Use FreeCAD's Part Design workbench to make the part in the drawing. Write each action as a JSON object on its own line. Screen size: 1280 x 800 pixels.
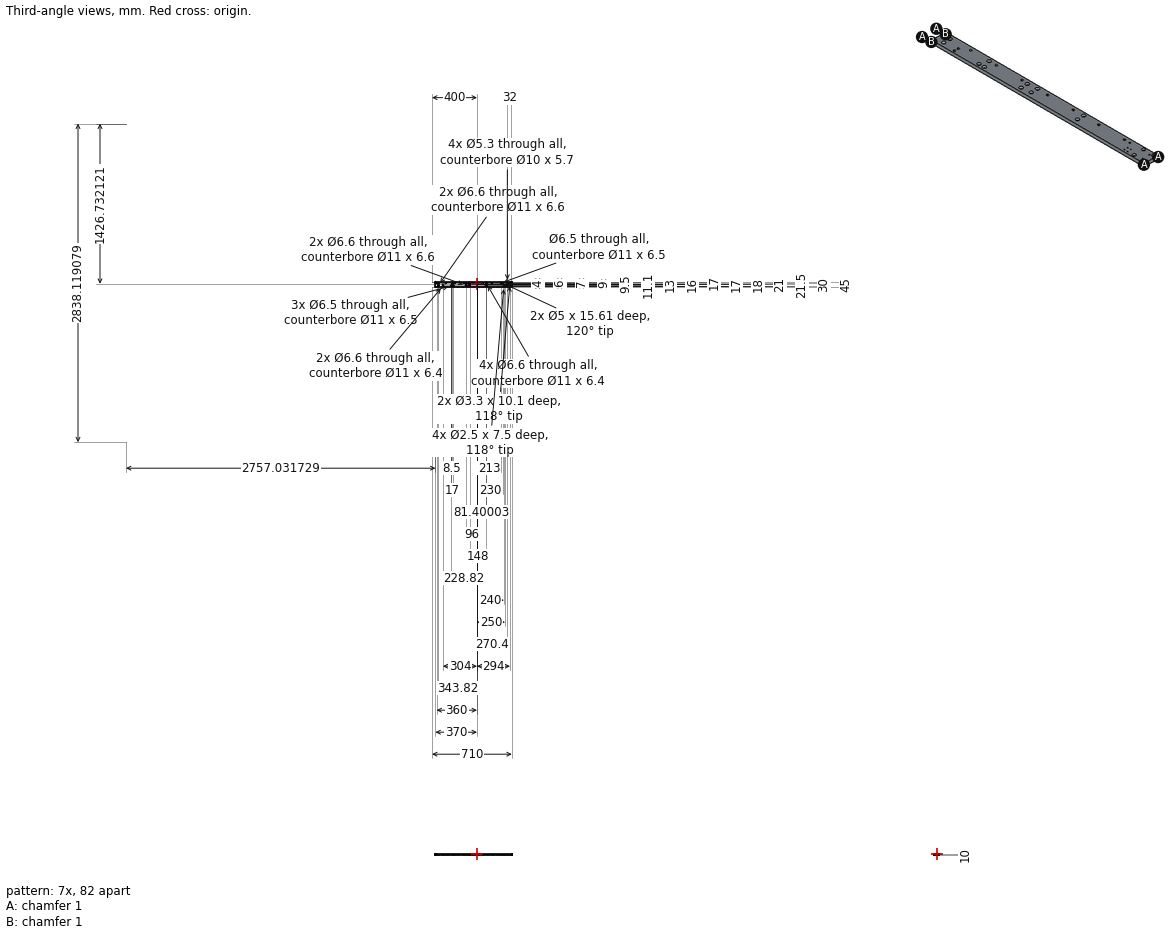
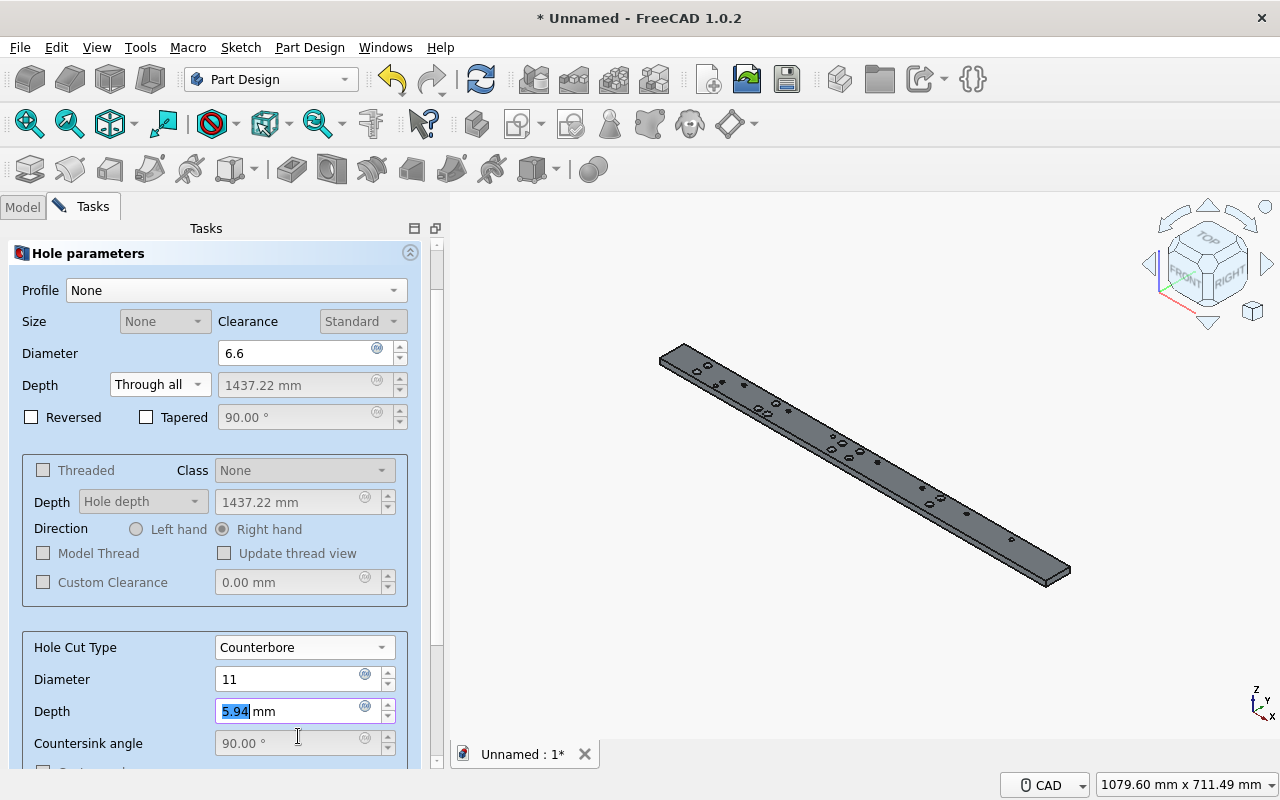
{"action": "type", "text": "6.4"}
{"action": "key", "text": "Tab"}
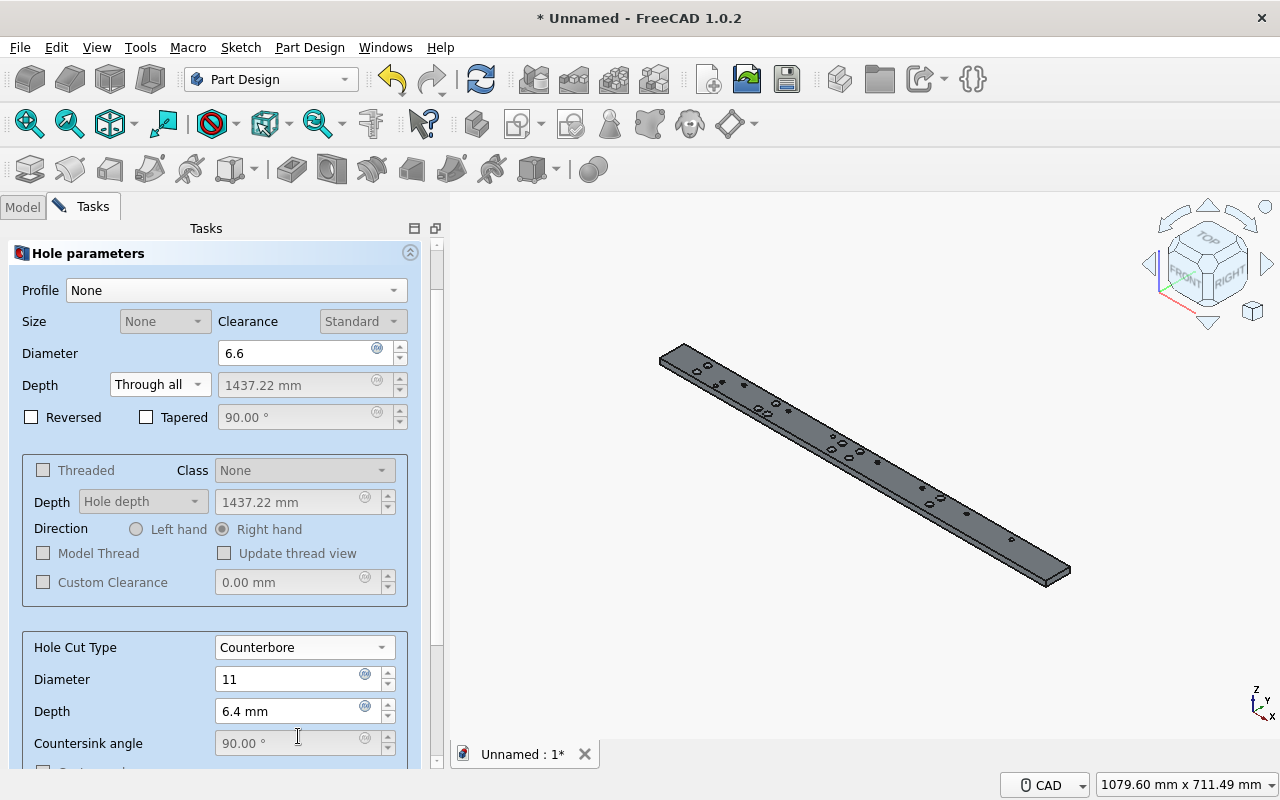
{"action": "scroll", "coordinate": [437, 503], "scroll_direction": "up", "scroll_amount": 2}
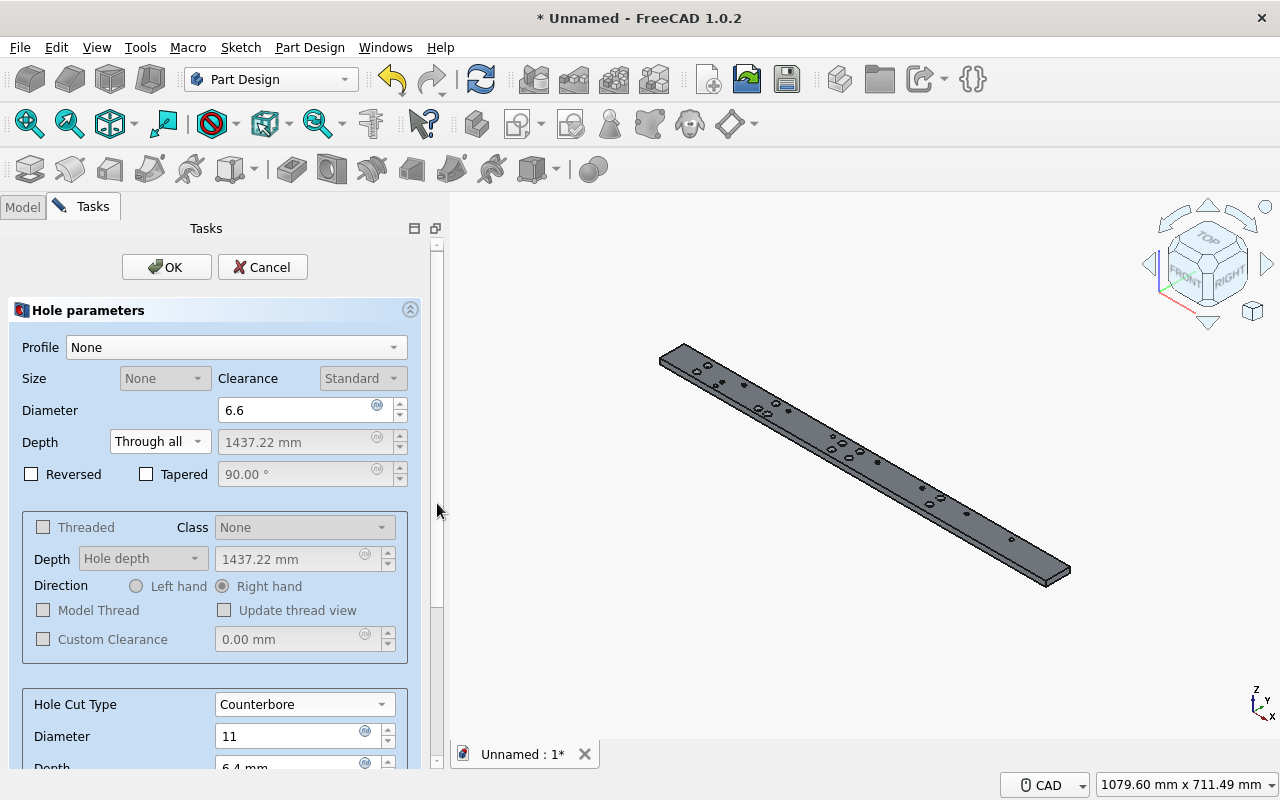
{"action": "left_click", "coordinate": [167, 267]}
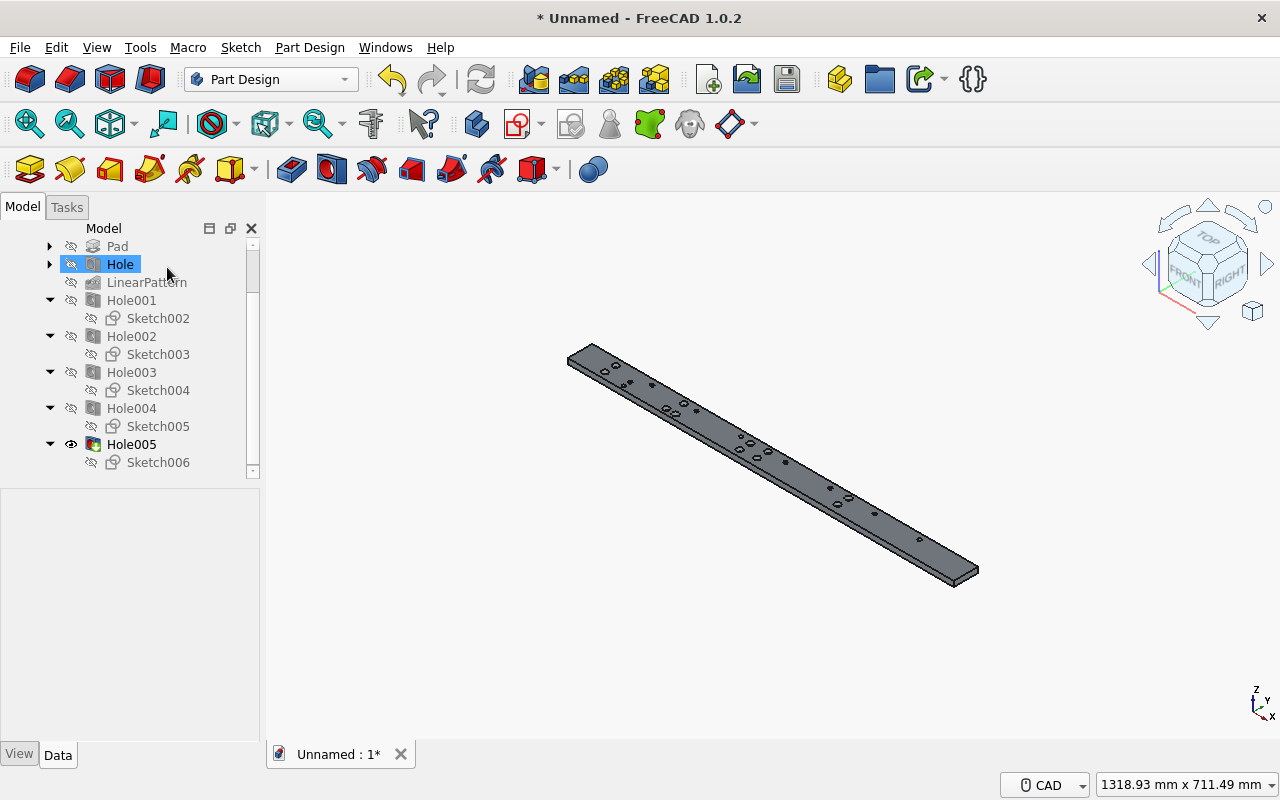
{"action": "left_click", "coordinate": [30, 124]}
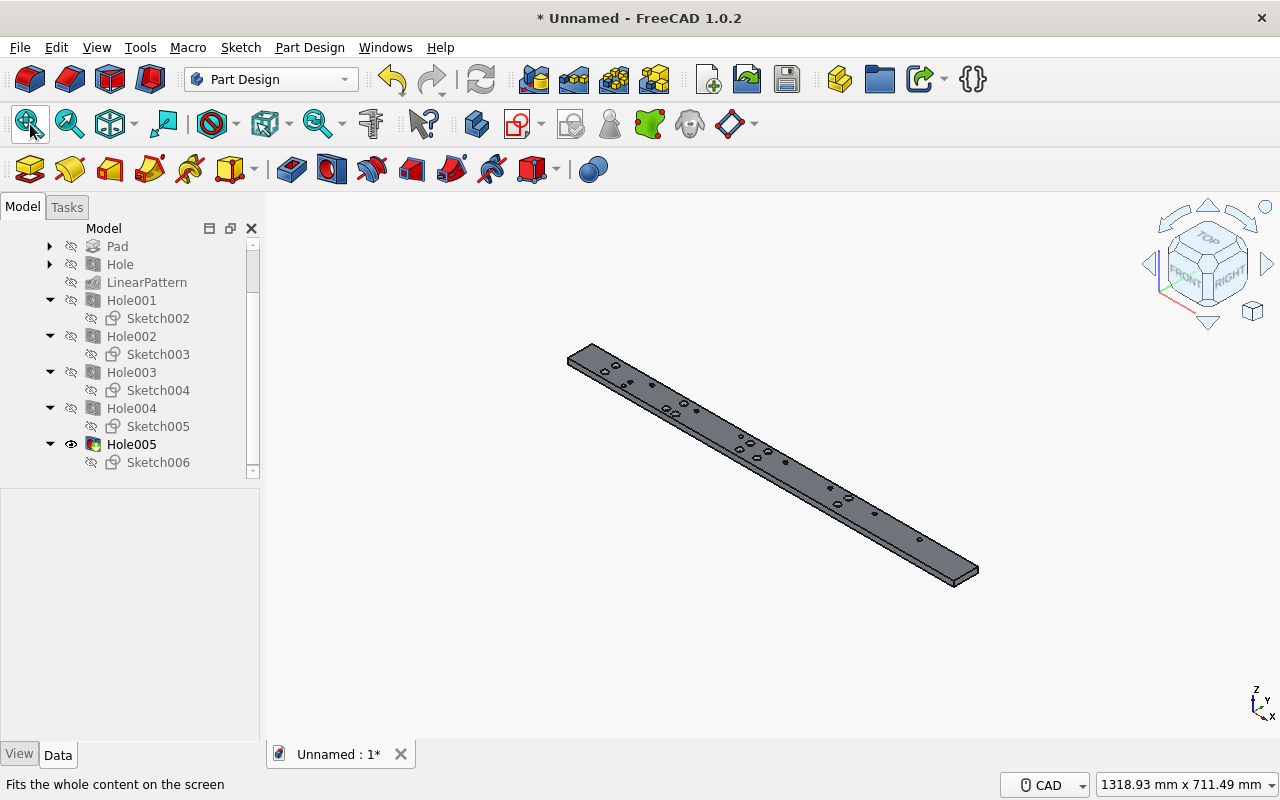
{"action": "scroll", "coordinate": [592, 346], "scroll_direction": "up", "scroll_amount": 9}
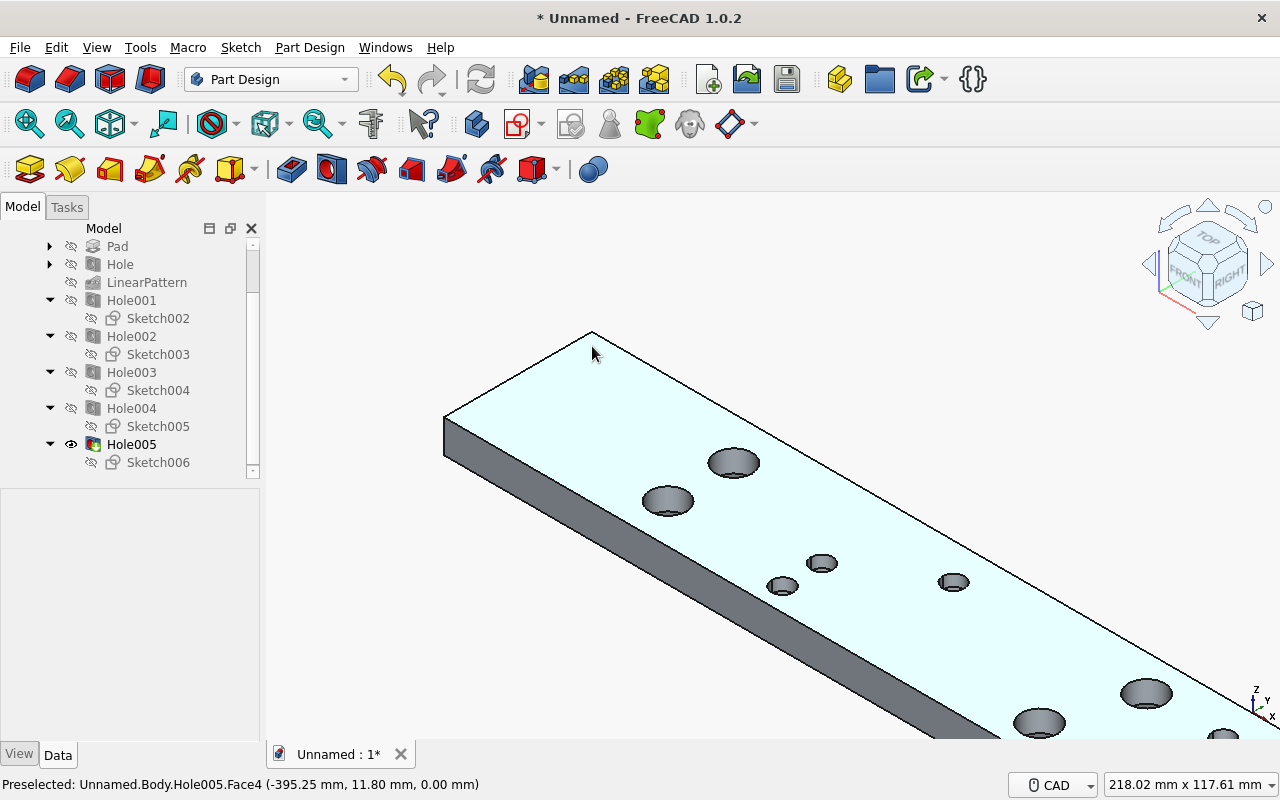
{"action": "left_click", "coordinate": [30, 124]}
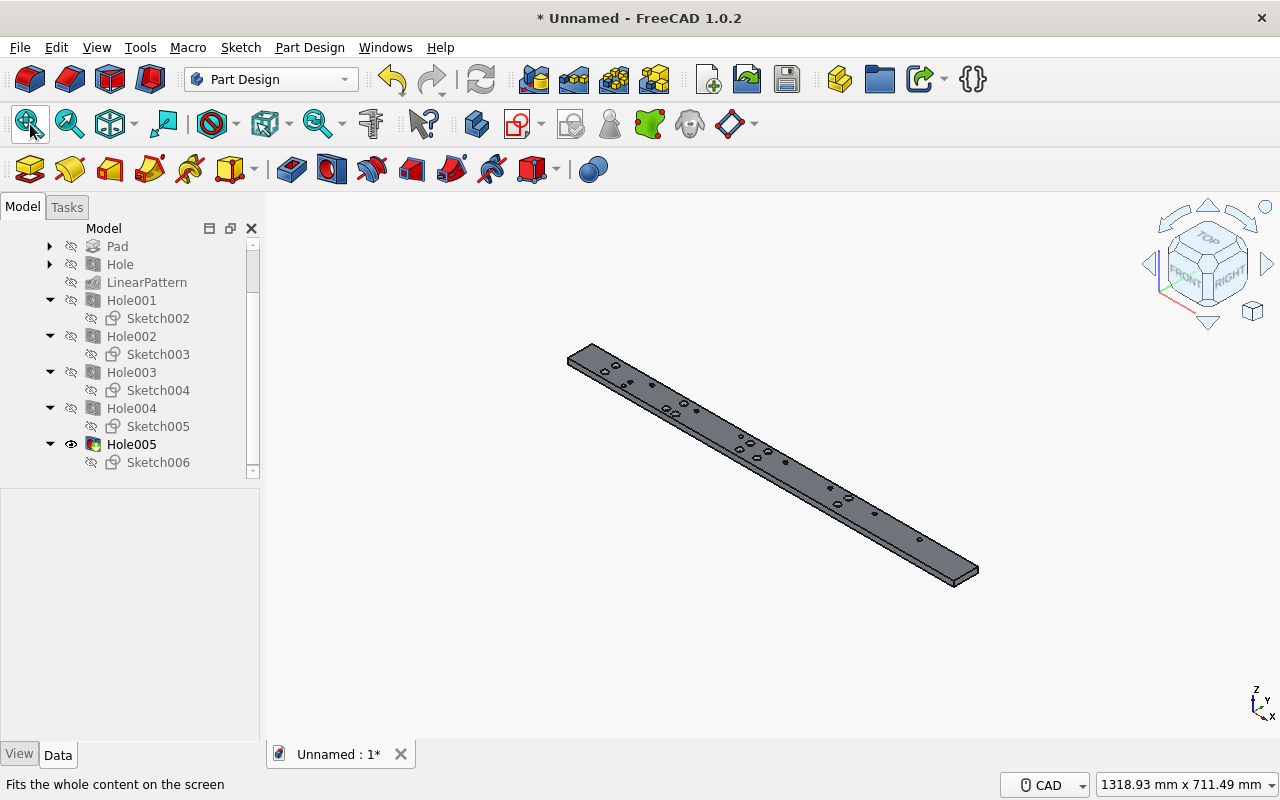
{"action": "key", "text": "2"}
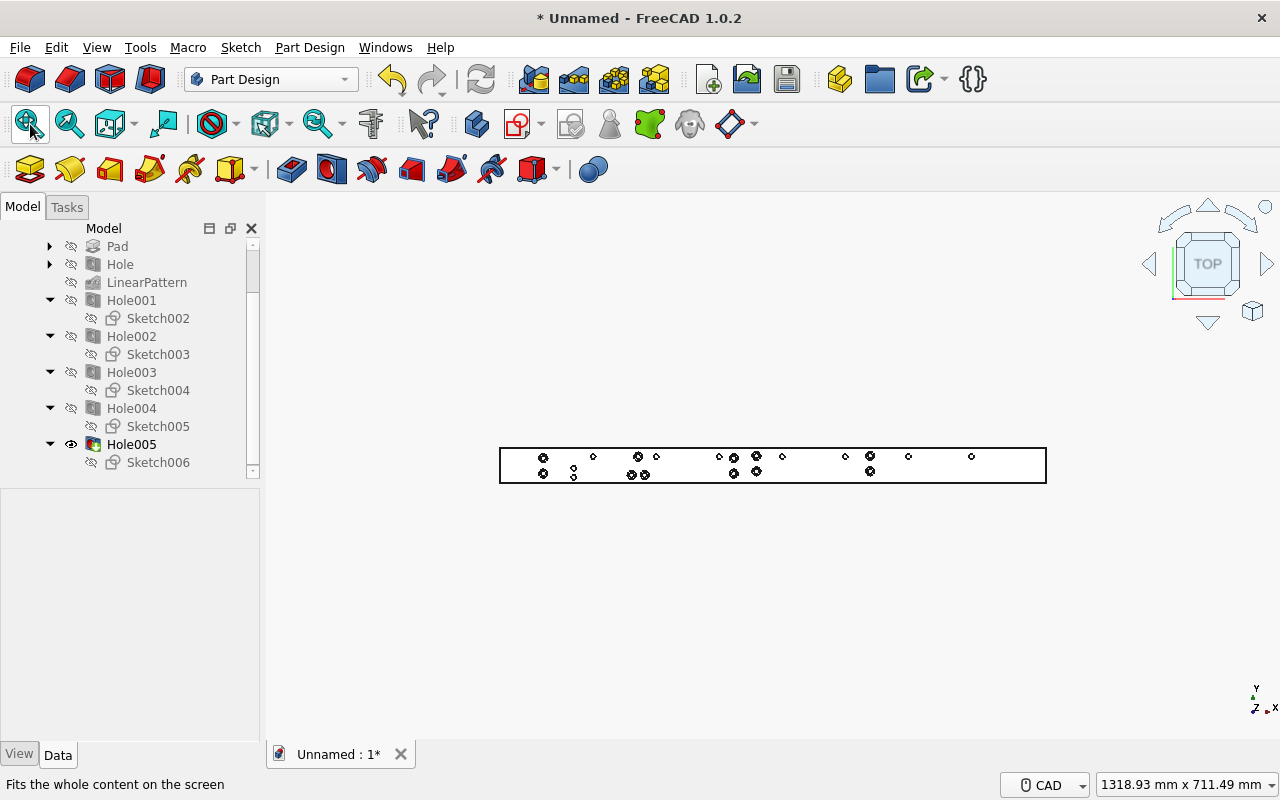
{"action": "scroll", "coordinate": [500, 447], "scroll_direction": "up", "scroll_amount": 9}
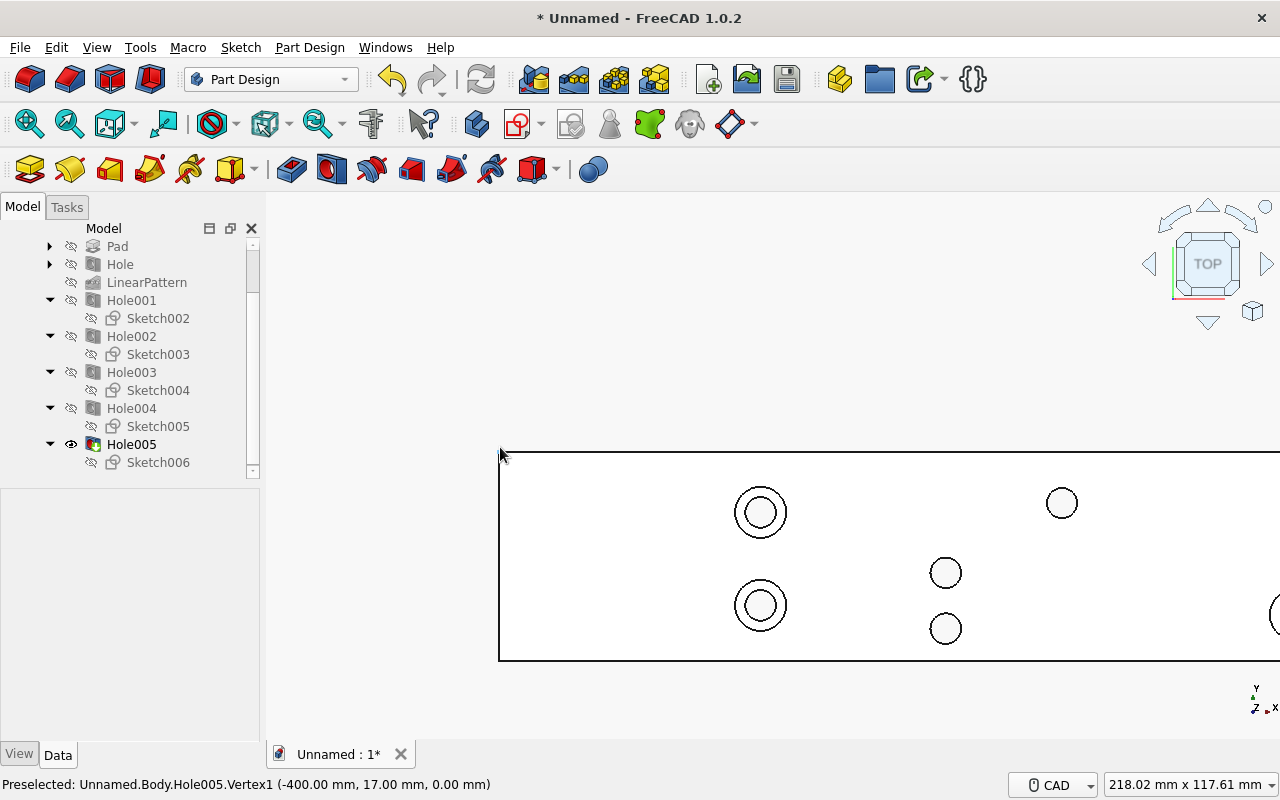
{"action": "left_click", "coordinate": [30, 124]}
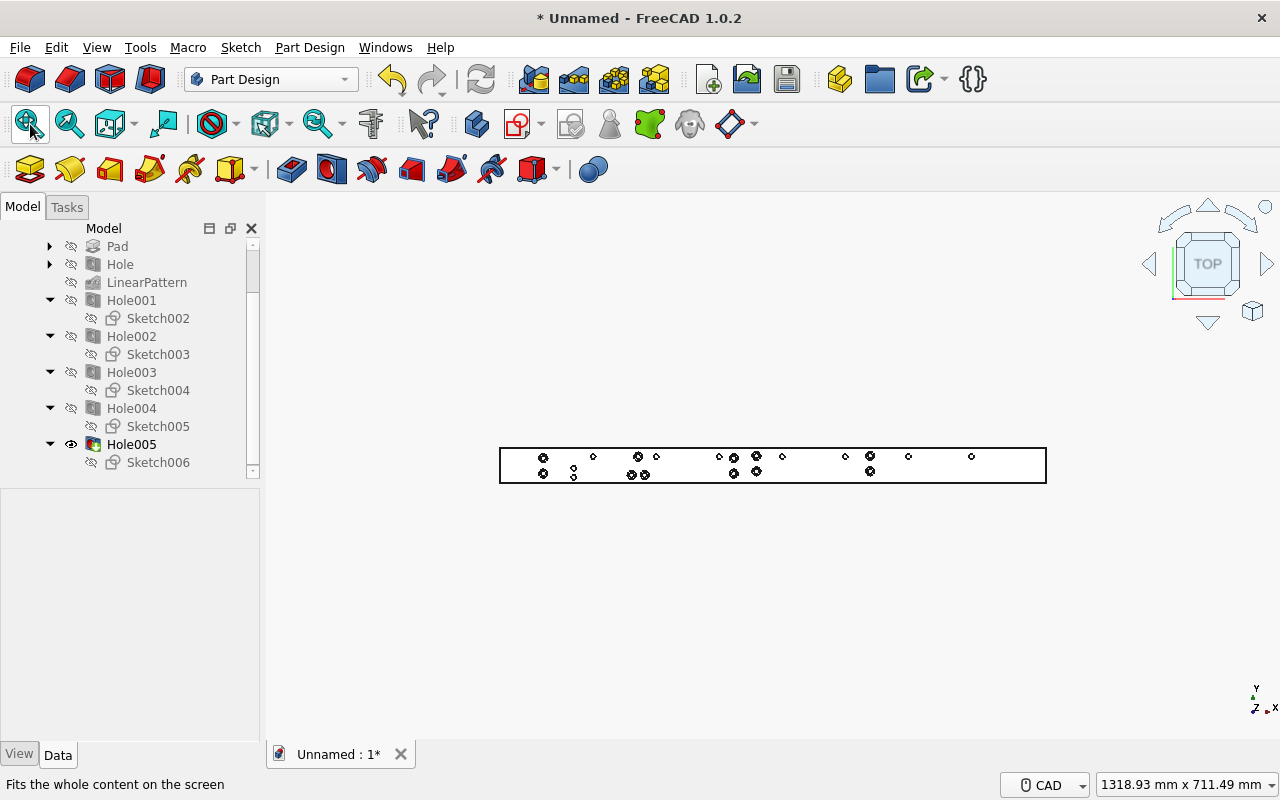
{"action": "key", "text": "0"}